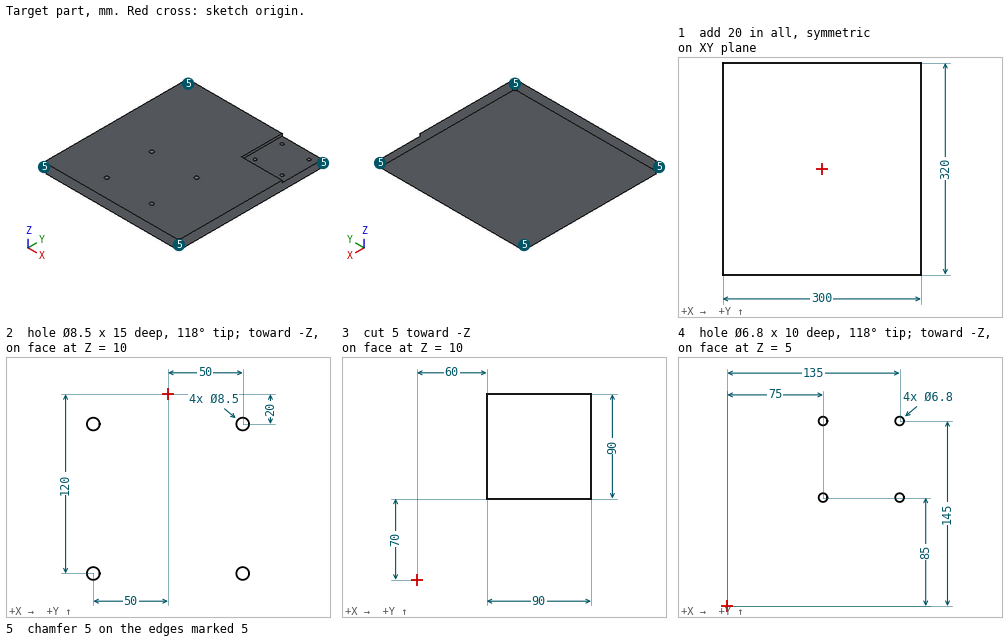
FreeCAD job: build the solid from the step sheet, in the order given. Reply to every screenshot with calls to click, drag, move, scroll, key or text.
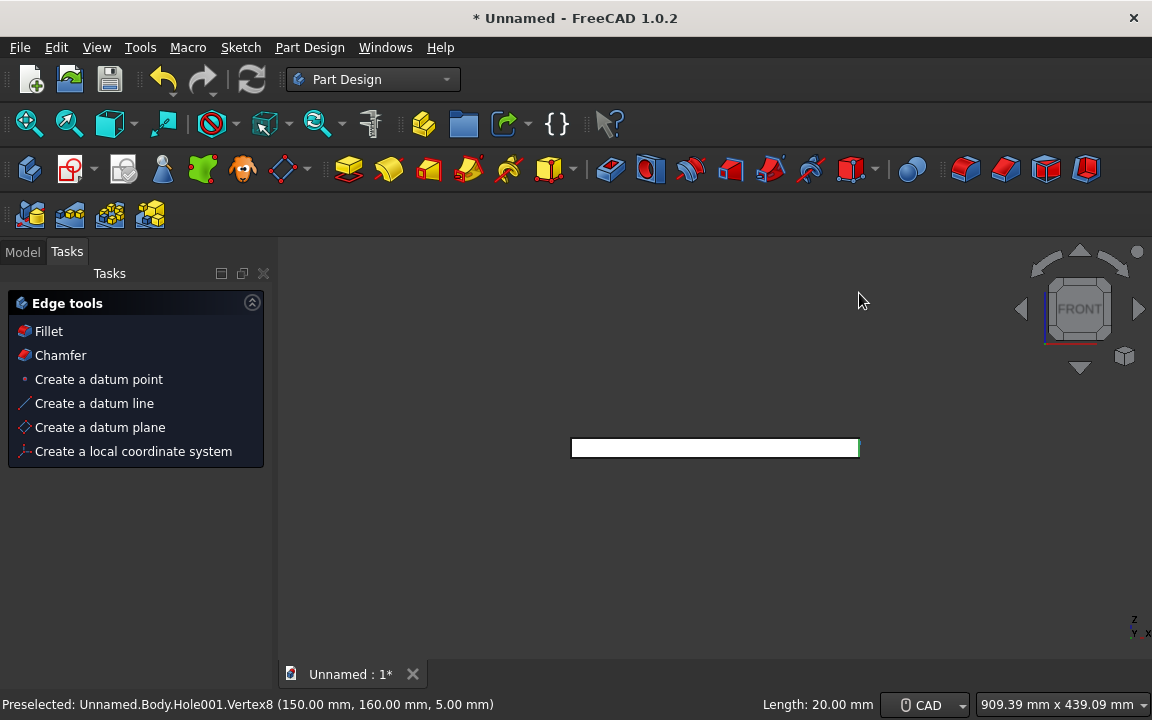
click(571, 447, ctrl)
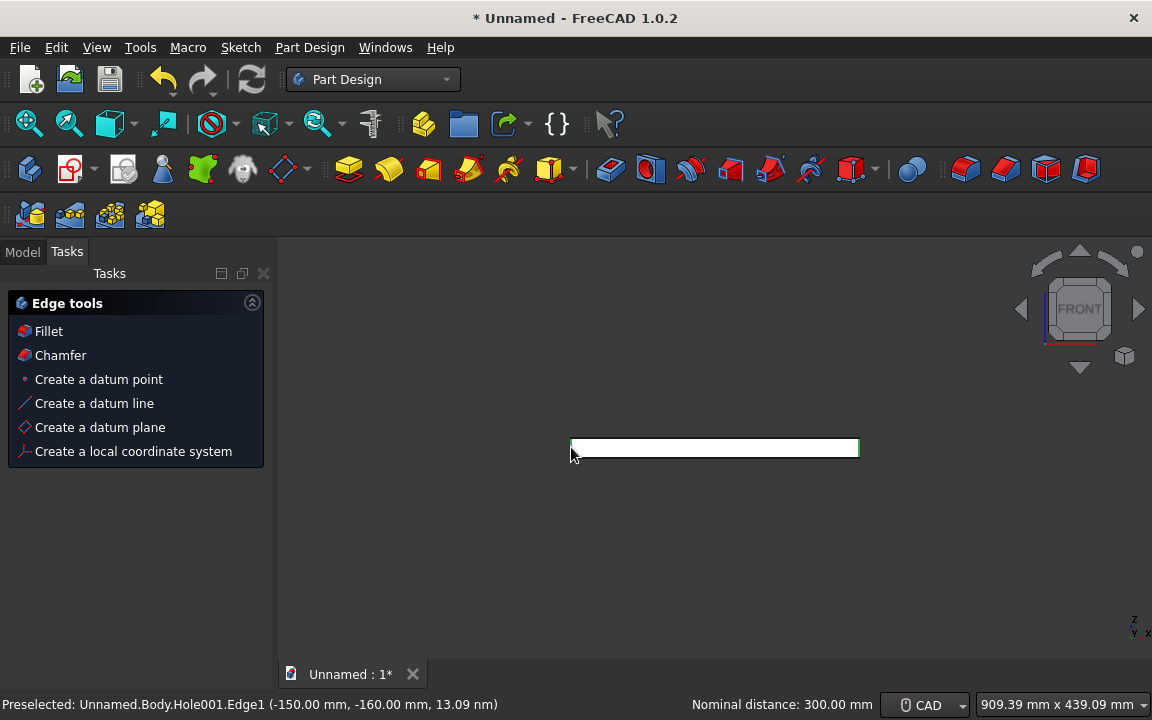
scroll(859, 449, up, 6)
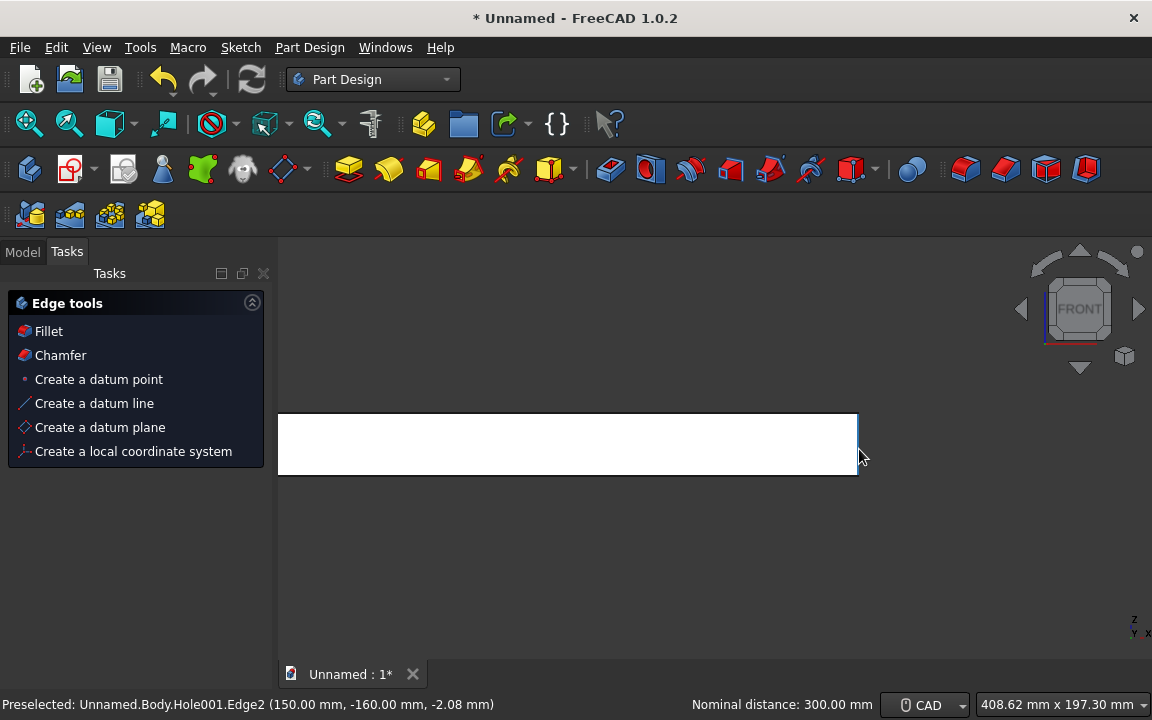
key(v)
key(f)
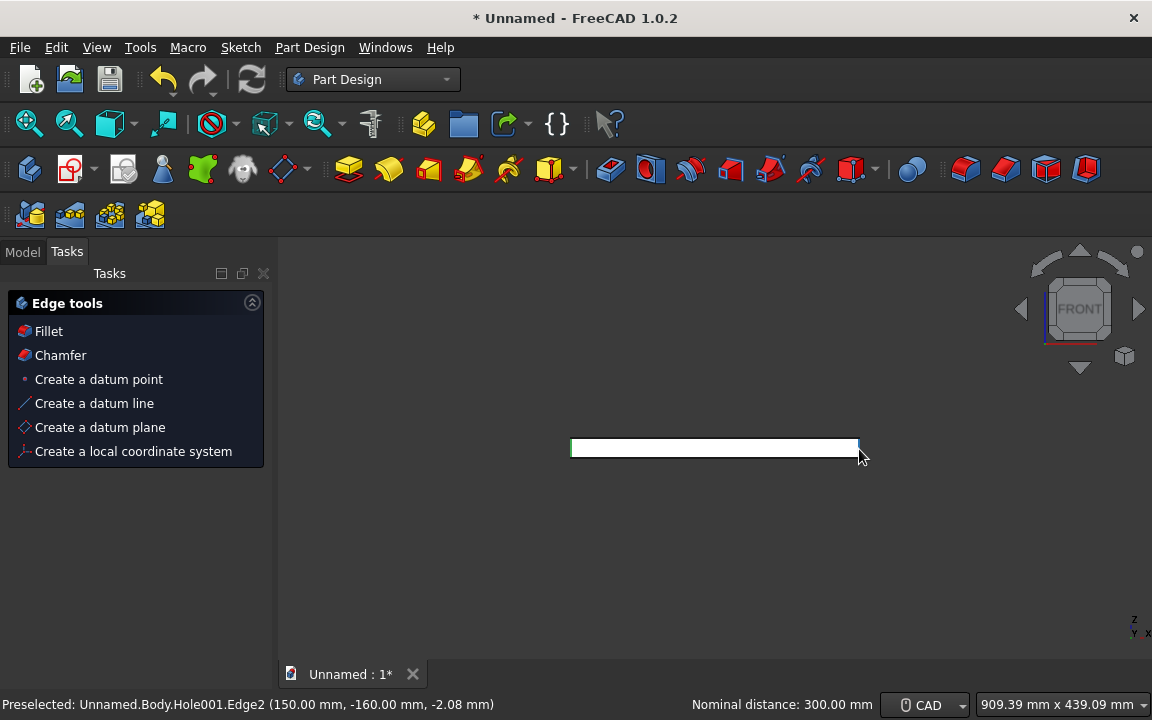
key(3)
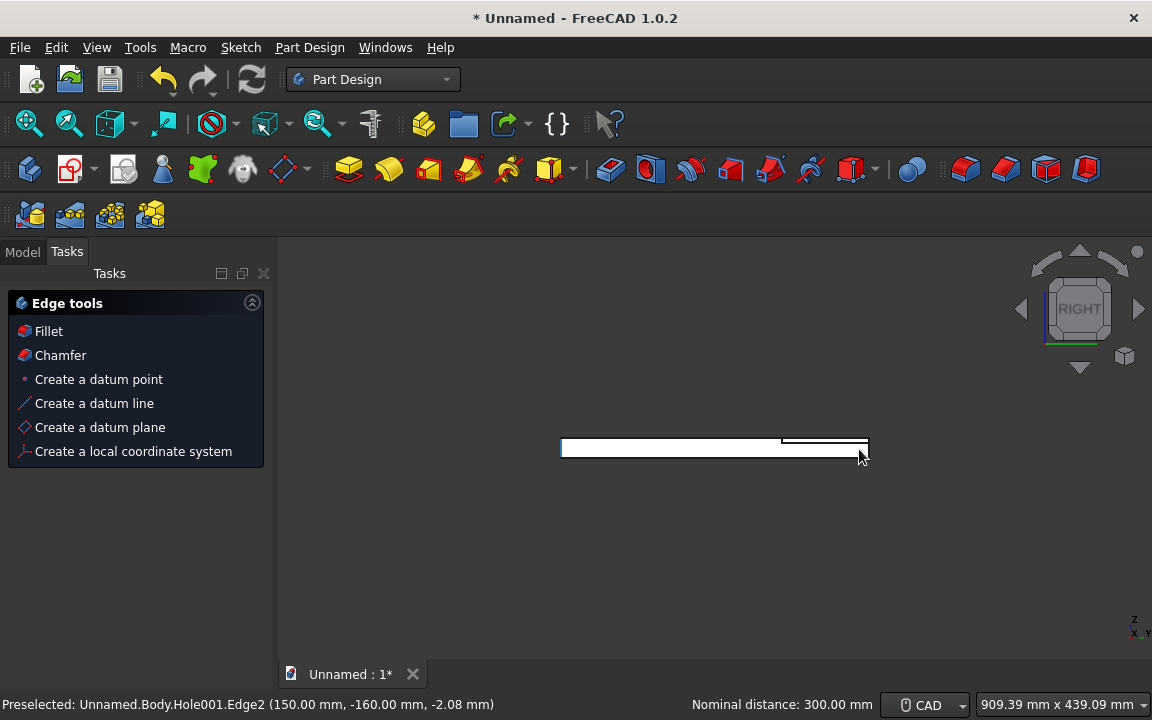
key(v)
key(f)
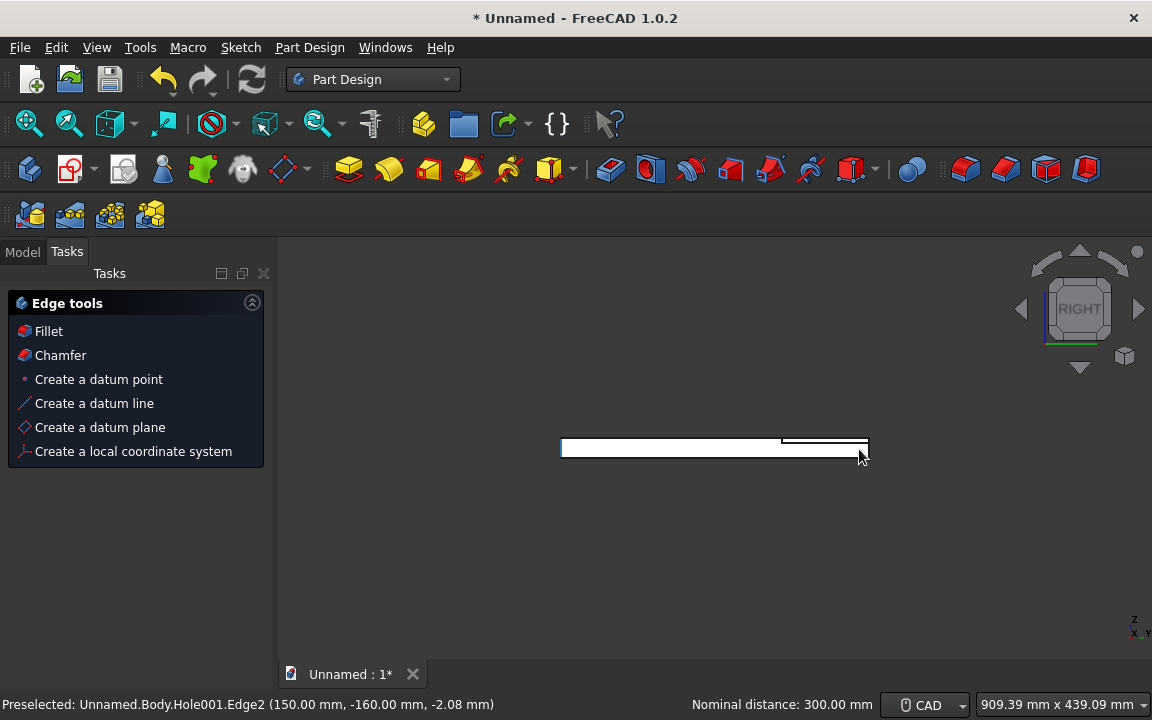
click(869, 449, ctrl)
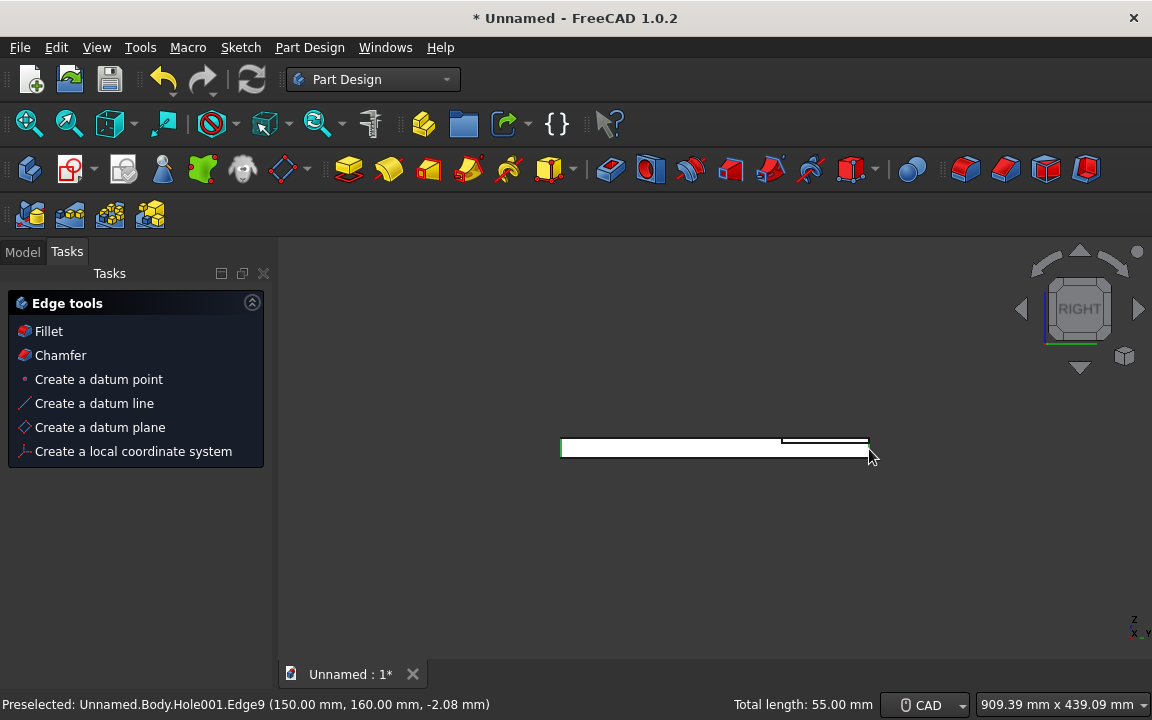
scroll(869, 447, up, 4)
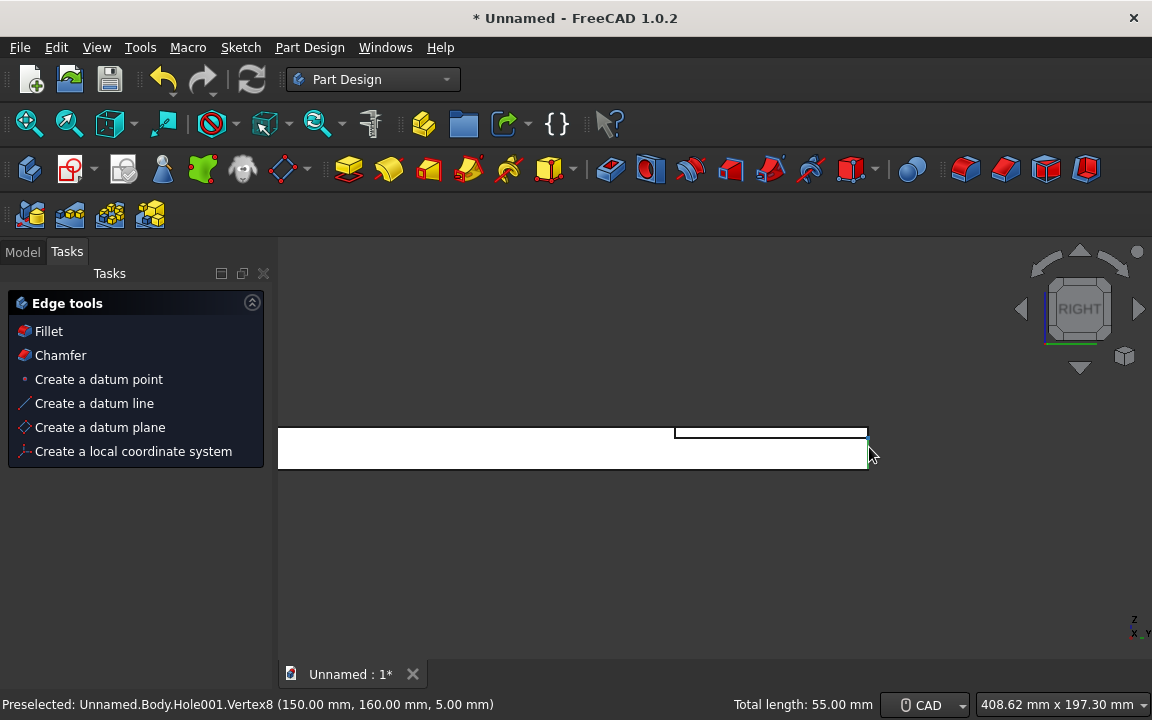
click(30, 124)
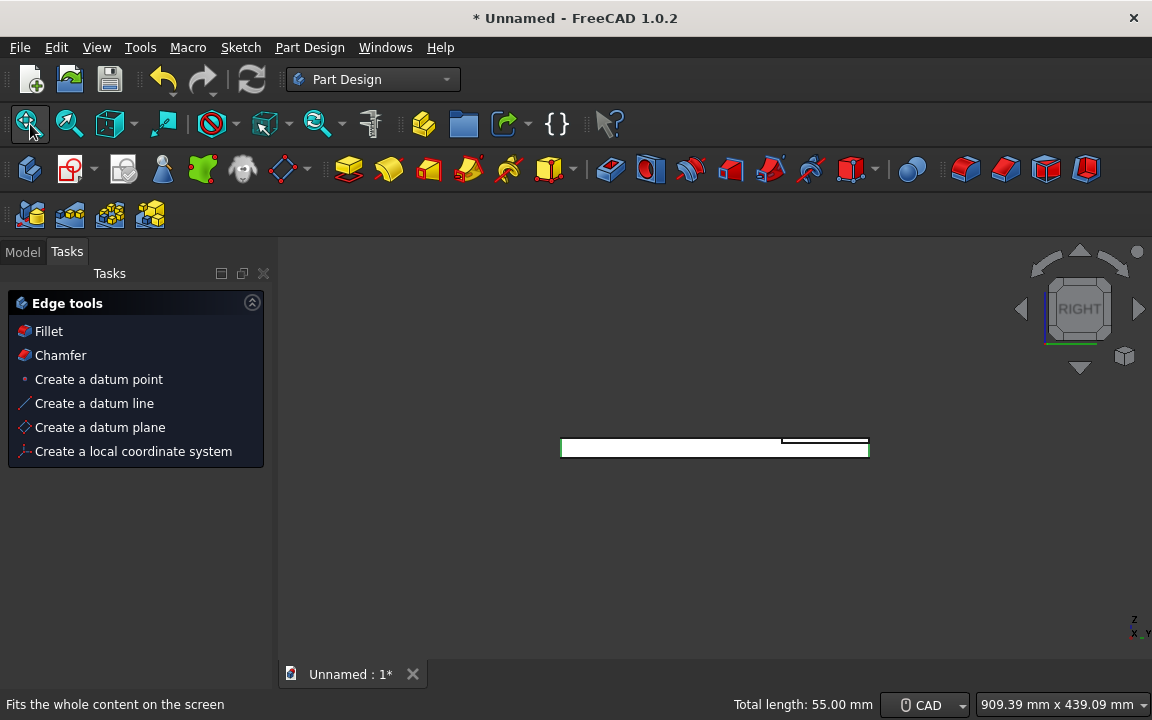
key(5)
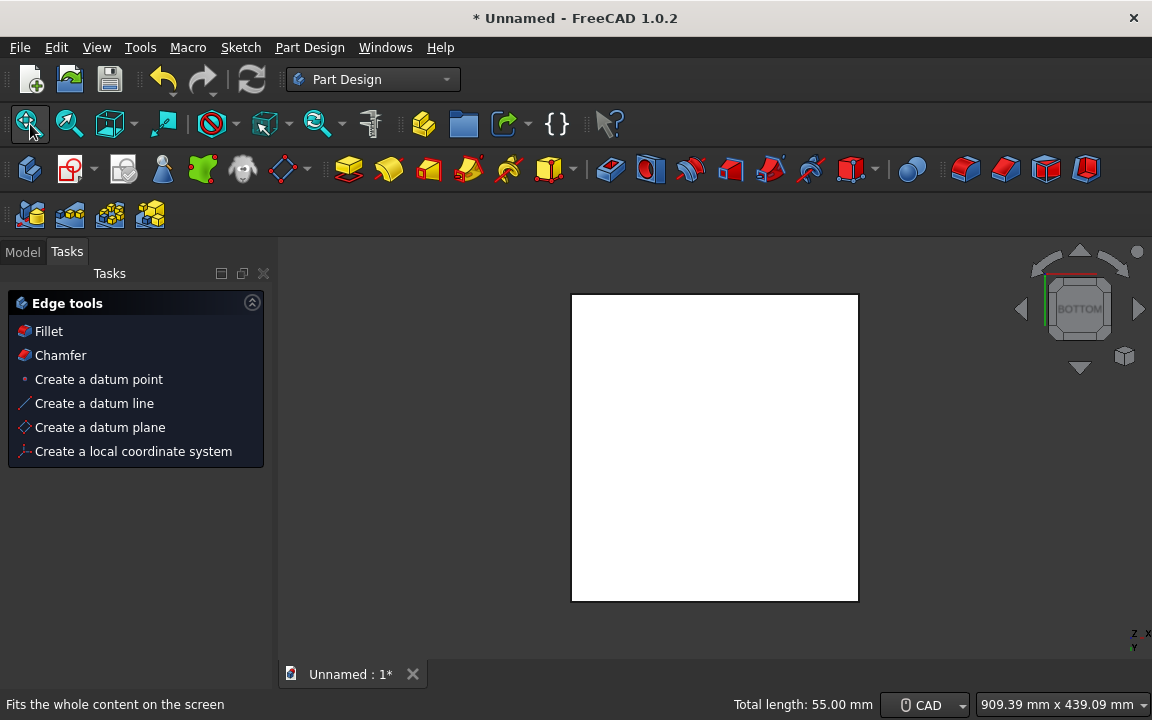
scroll(571, 601, up, 4)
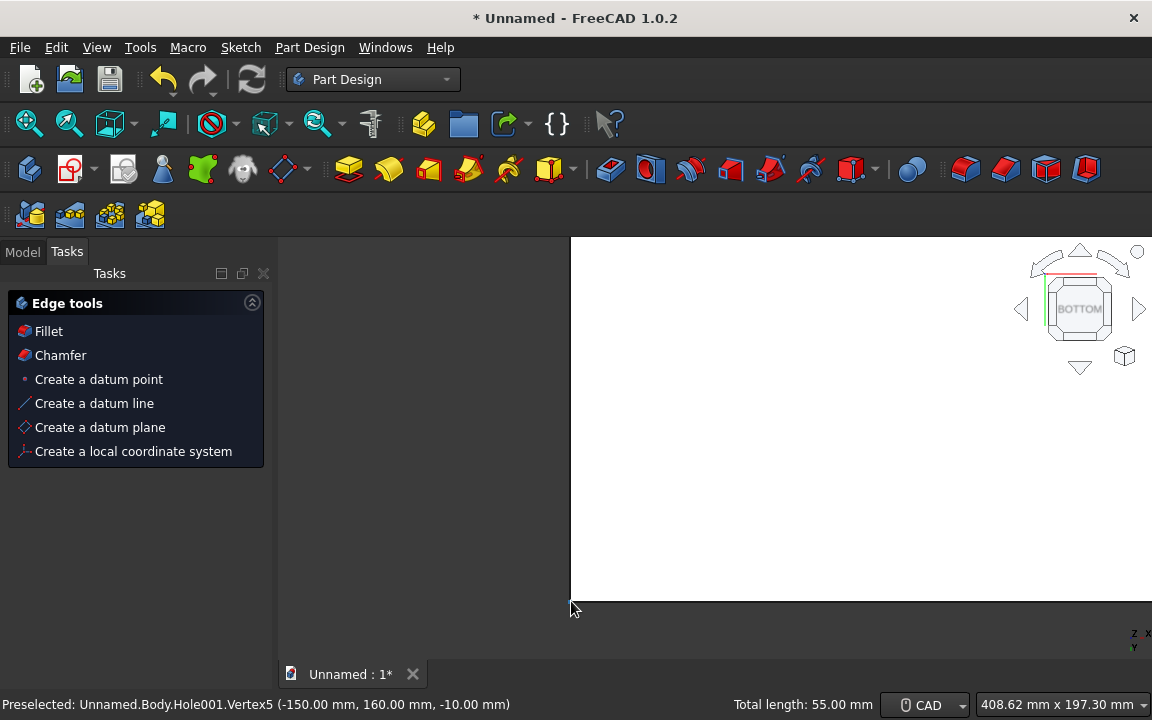
key(v)
key(f)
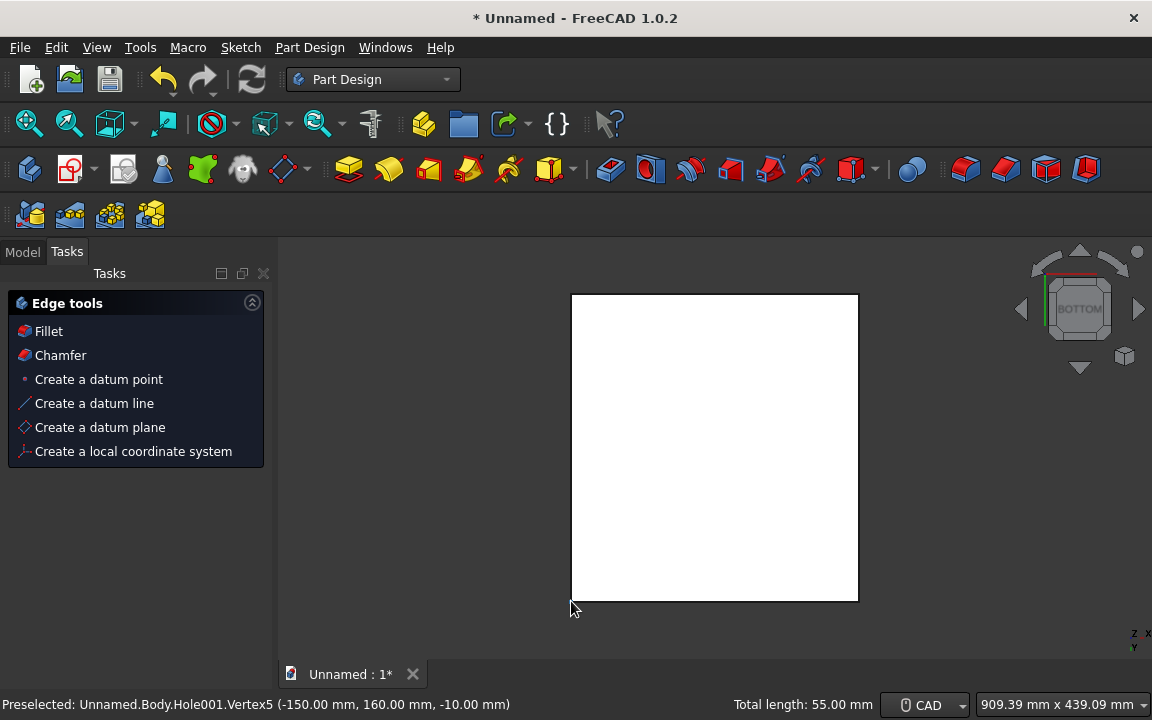
key(4)